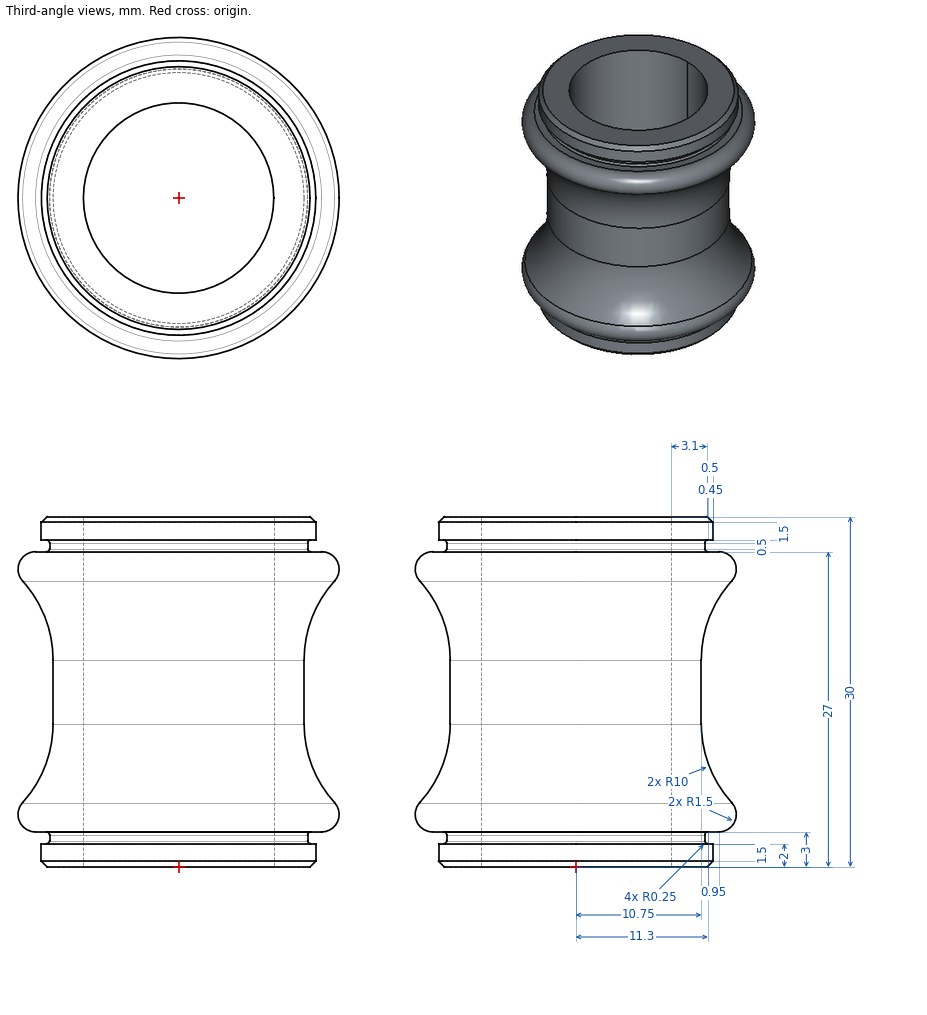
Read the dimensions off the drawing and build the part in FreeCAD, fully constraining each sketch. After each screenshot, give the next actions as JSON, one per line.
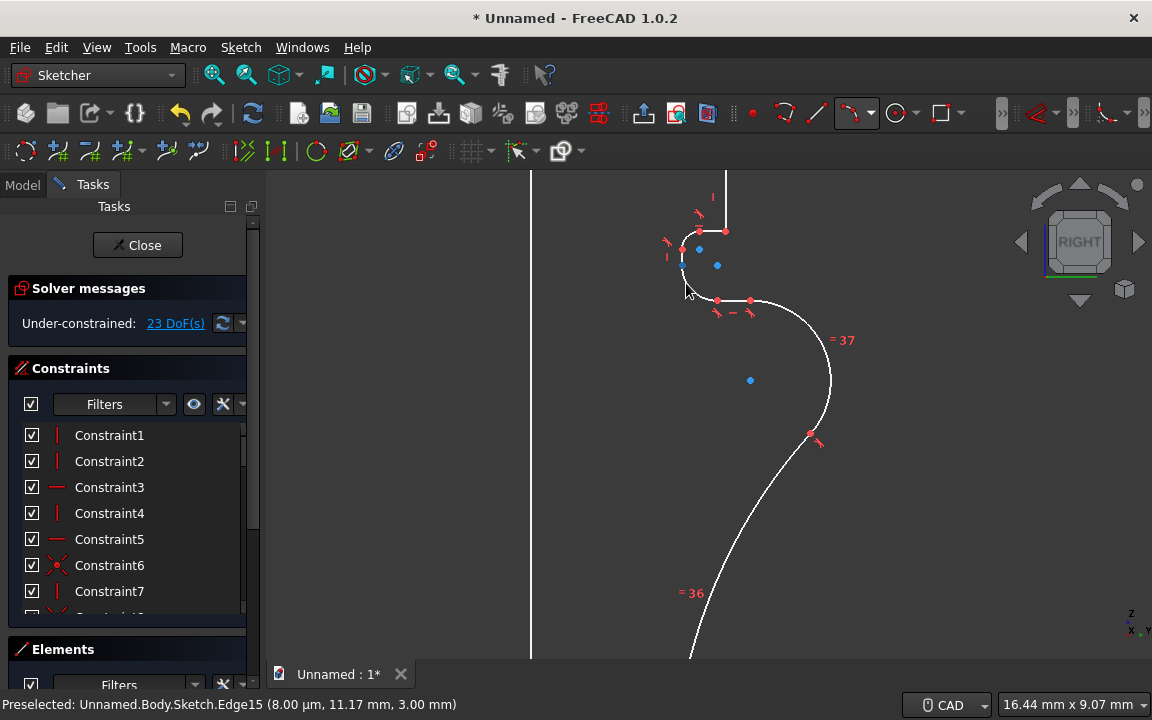
{"action": "left_click", "coordinate": [686, 282]}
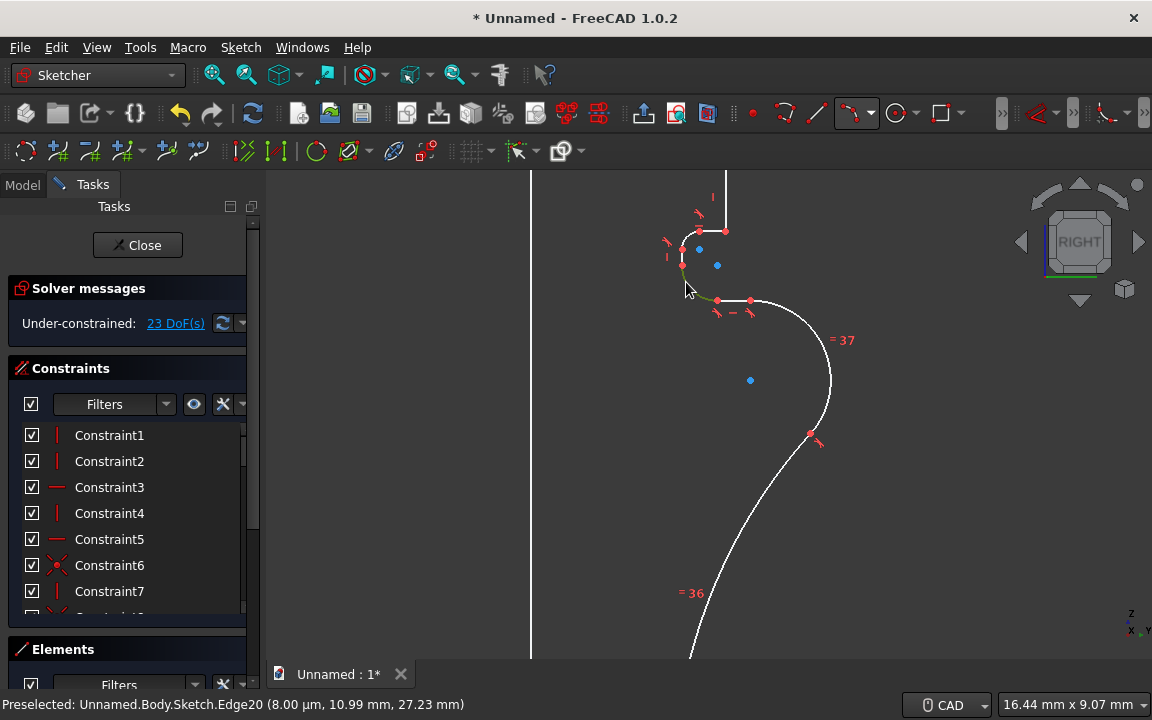
{"action": "left_click", "coordinate": [687, 237]}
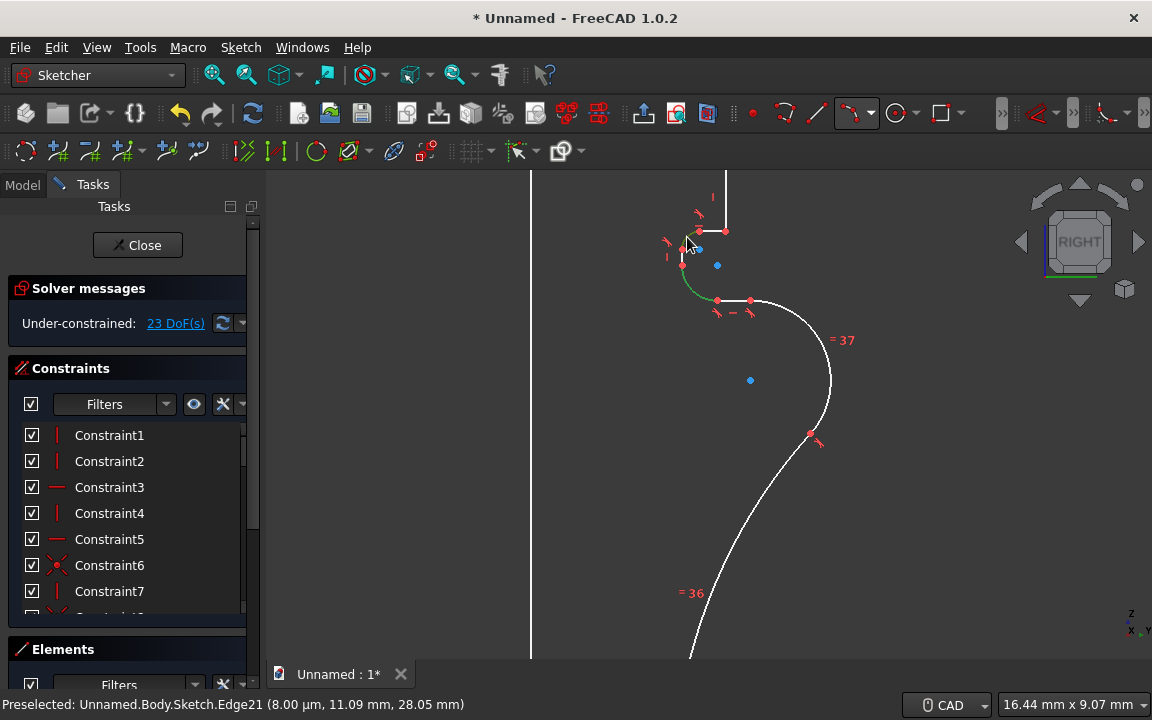
{"action": "scroll", "coordinate": [686, 282], "scroll_direction": "down", "scroll_amount": 8}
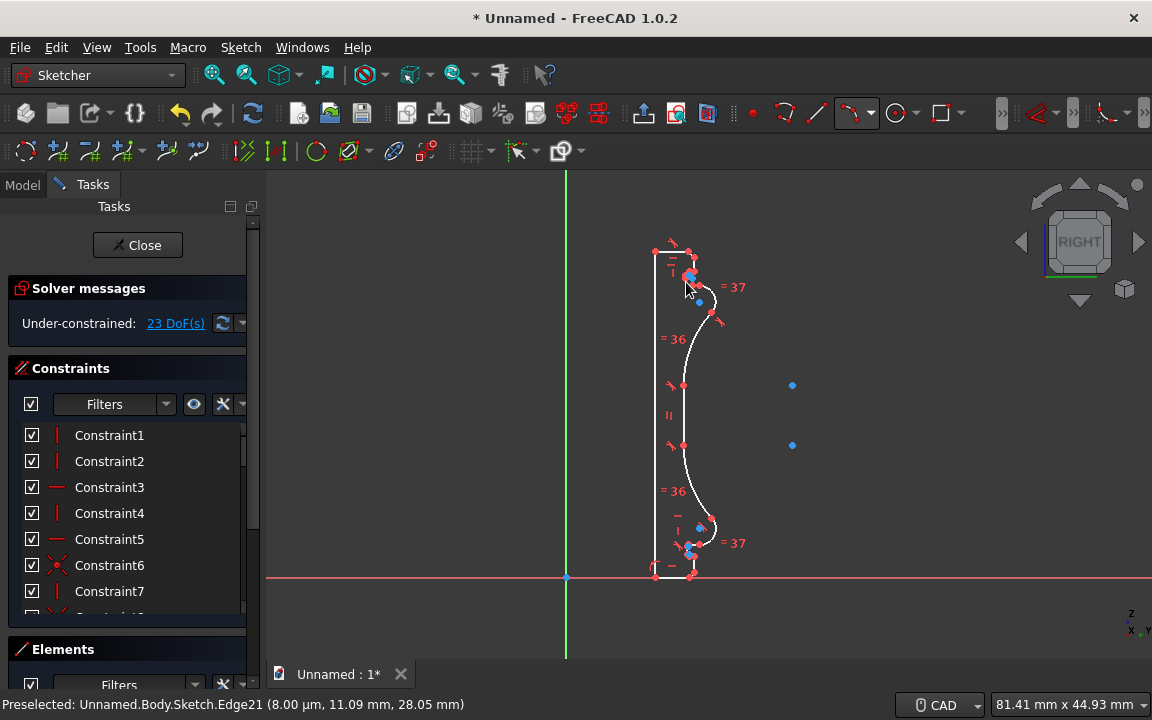
{"action": "scroll", "coordinate": [688, 556], "scroll_direction": "up", "scroll_amount": 11}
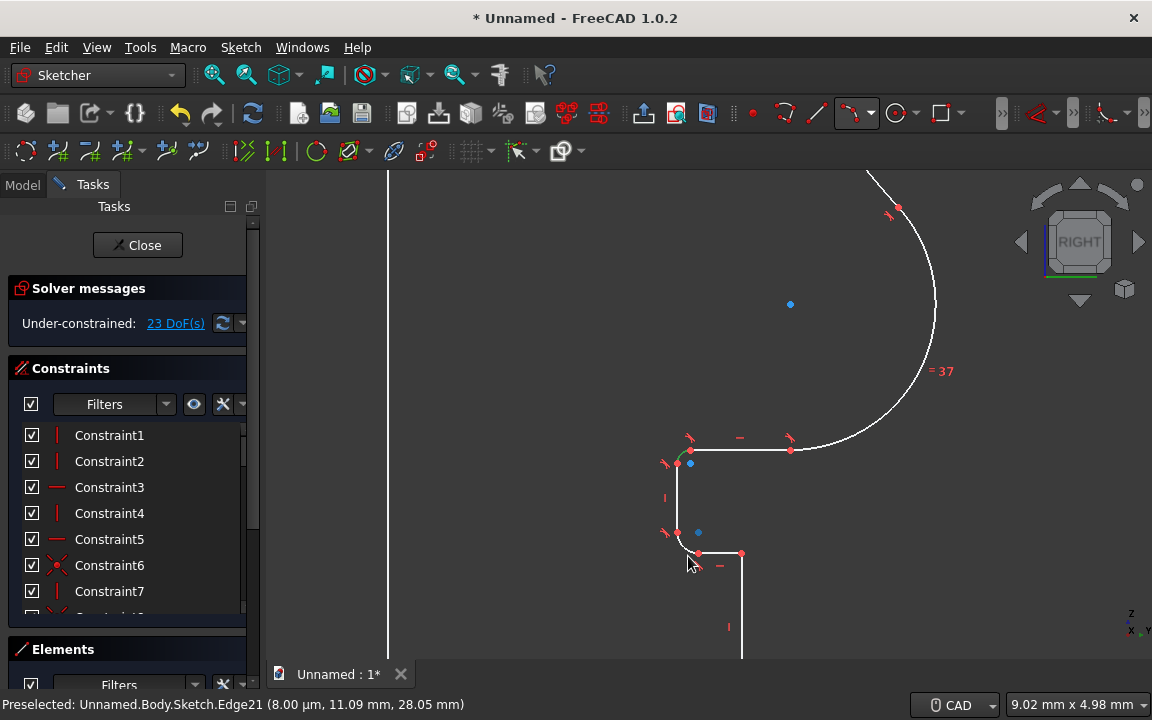
{"action": "left_click", "coordinate": [684, 547]}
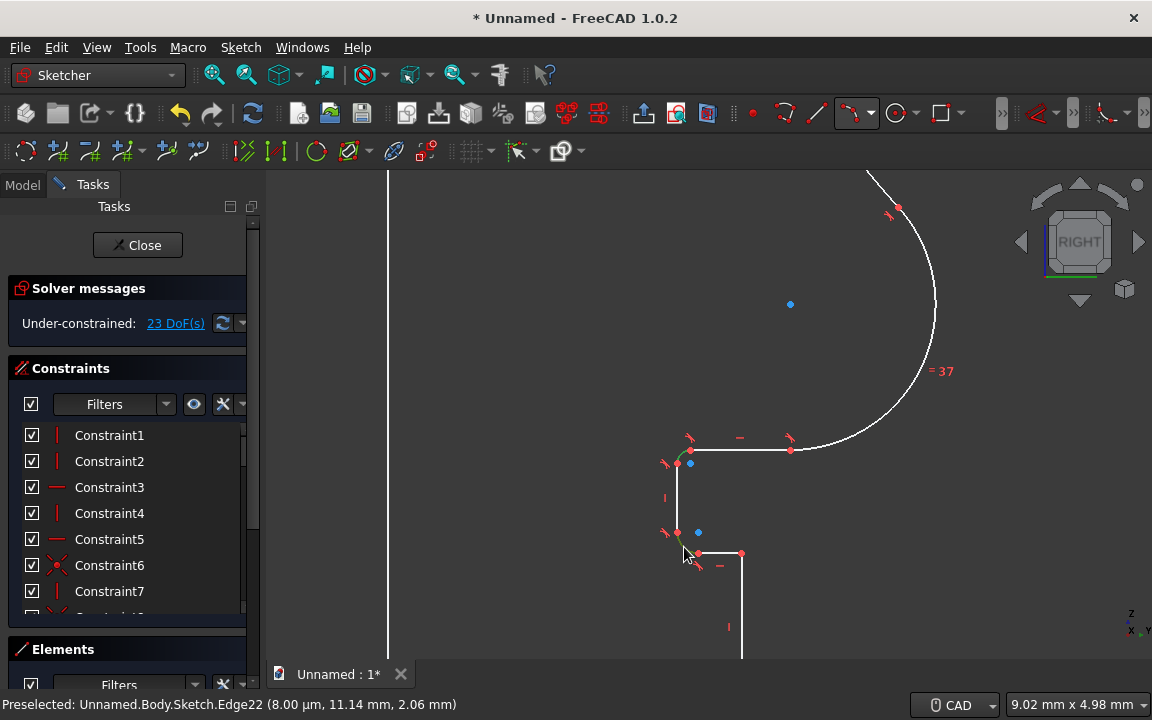
{"action": "key", "text": "e"}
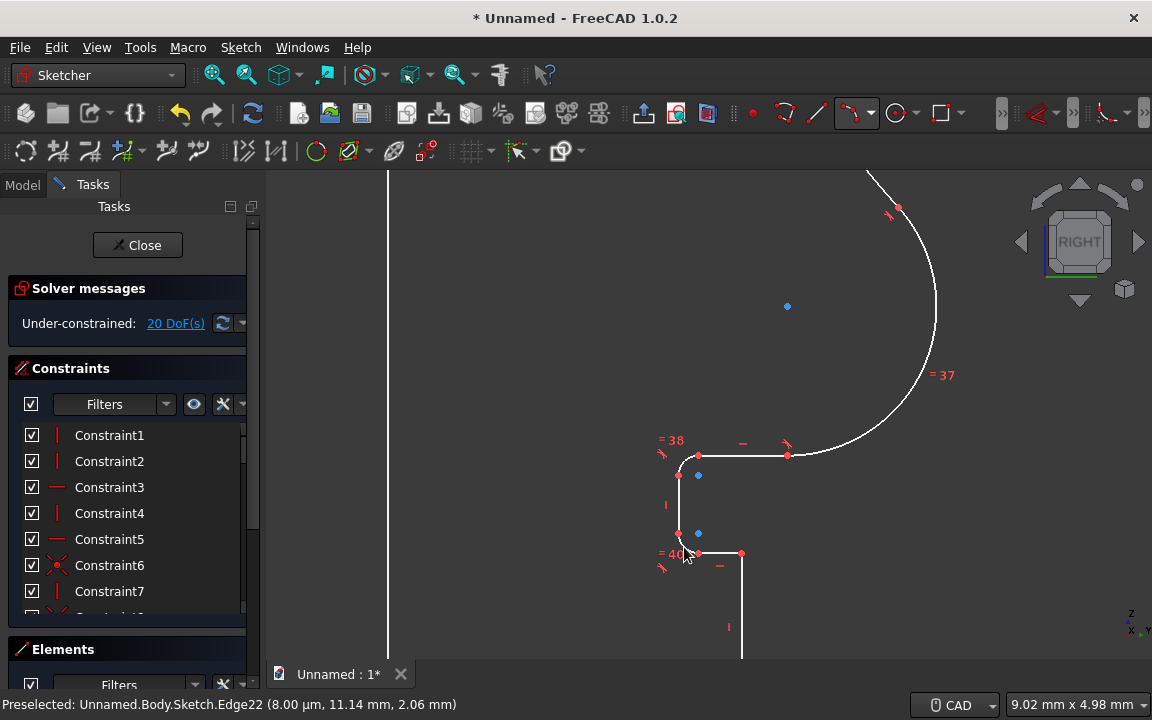
{"action": "left_click", "coordinate": [1036, 114]}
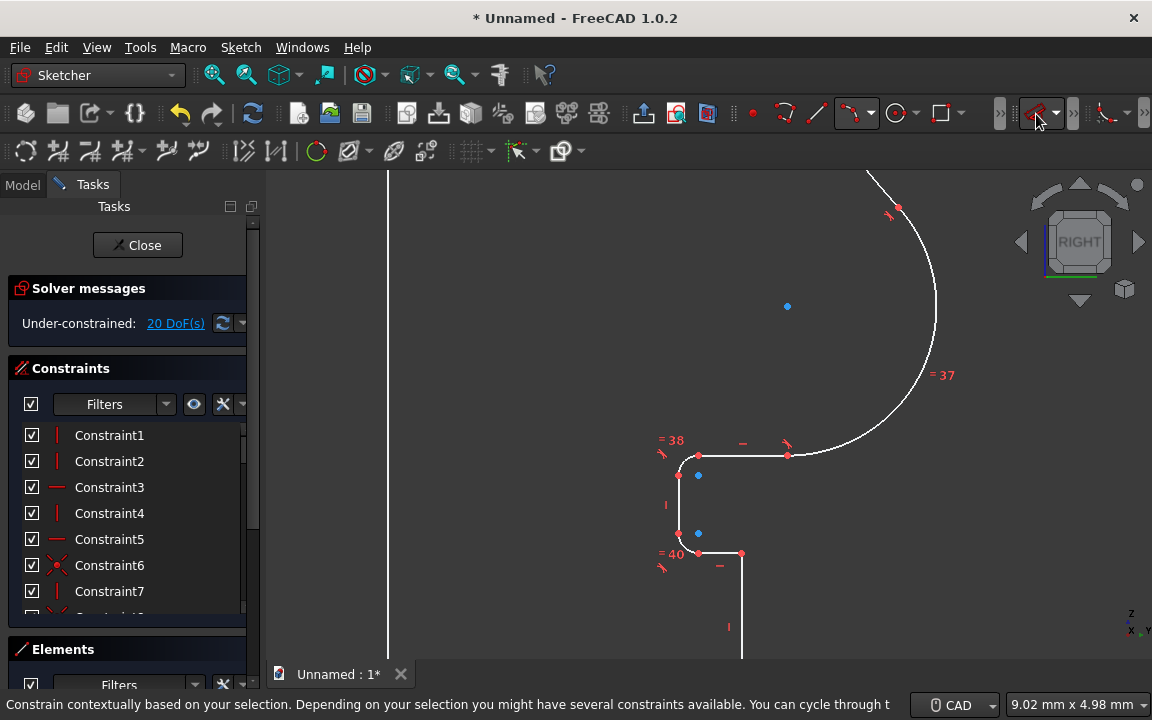
{"action": "scroll", "coordinate": [689, 458], "scroll_direction": "up", "scroll_amount": 3}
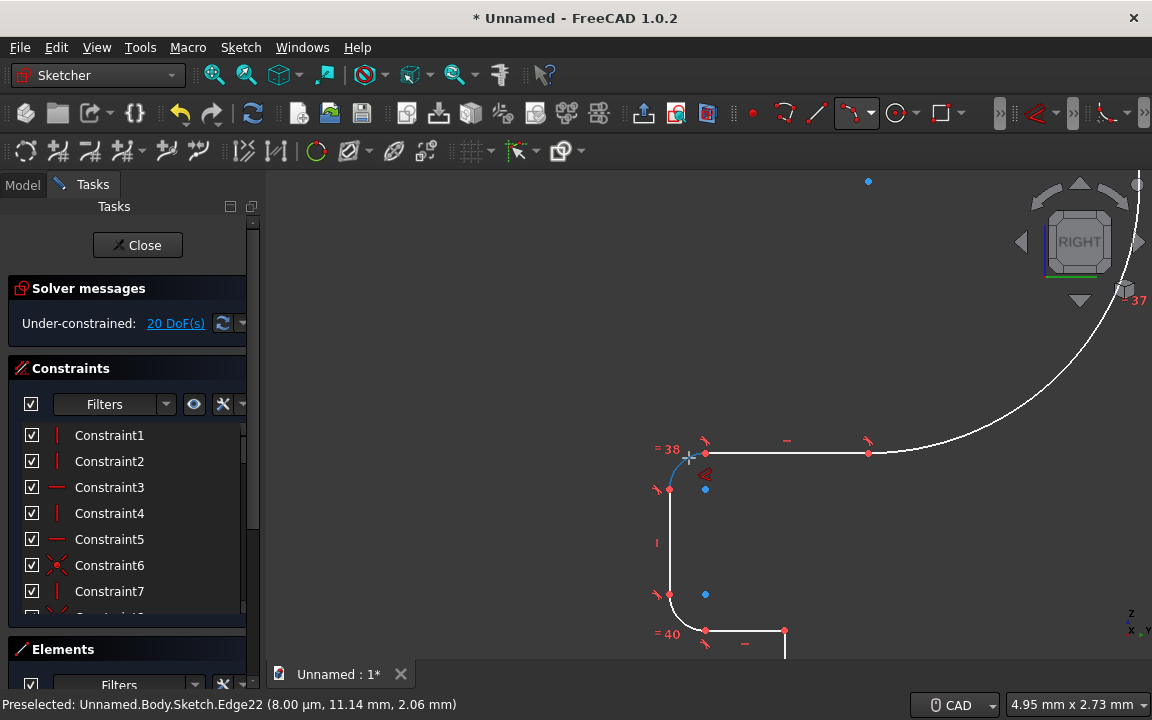
{"action": "left_click", "coordinate": [689, 457]}
{"action": "left_click", "coordinate": [674, 429]}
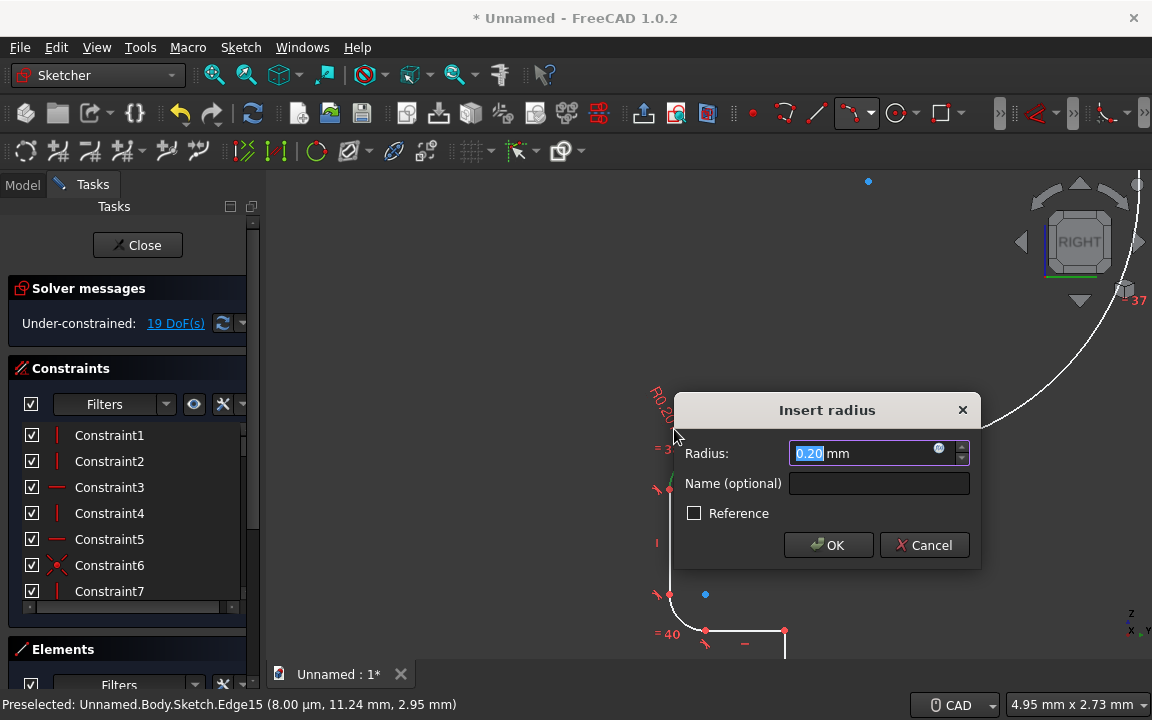
{"action": "type", "text": "0.25"}
{"action": "key", "text": "Return"}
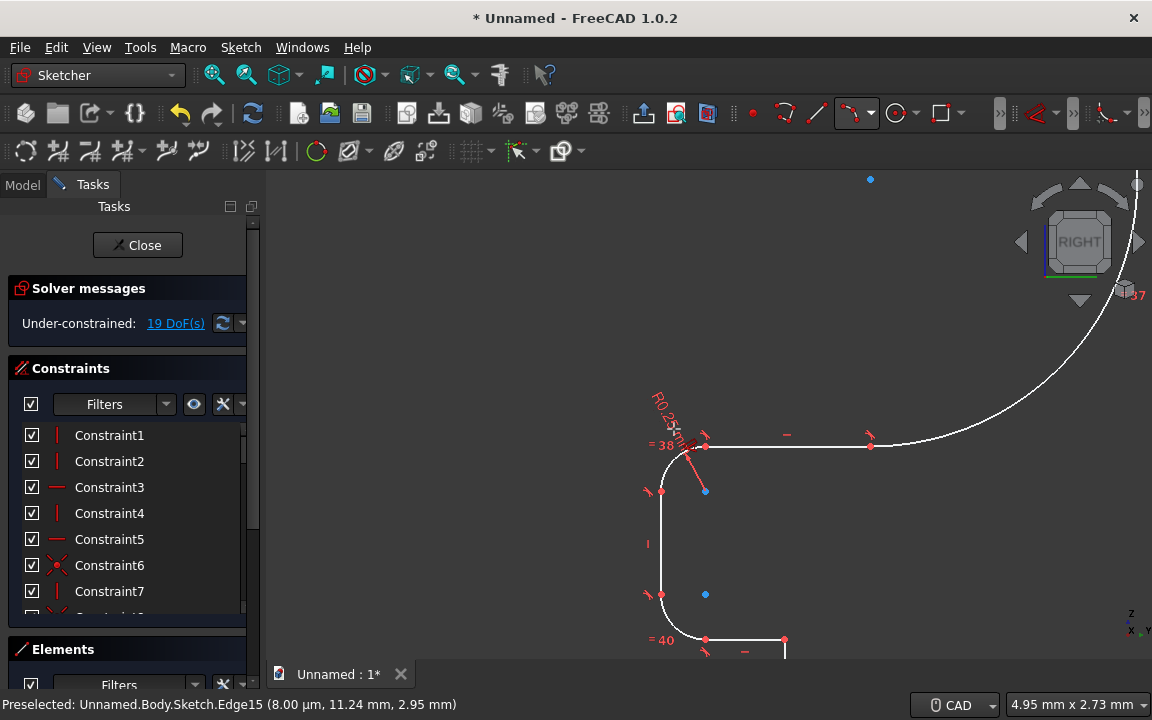
{"action": "scroll", "coordinate": [688, 551], "scroll_direction": "down", "scroll_amount": 14}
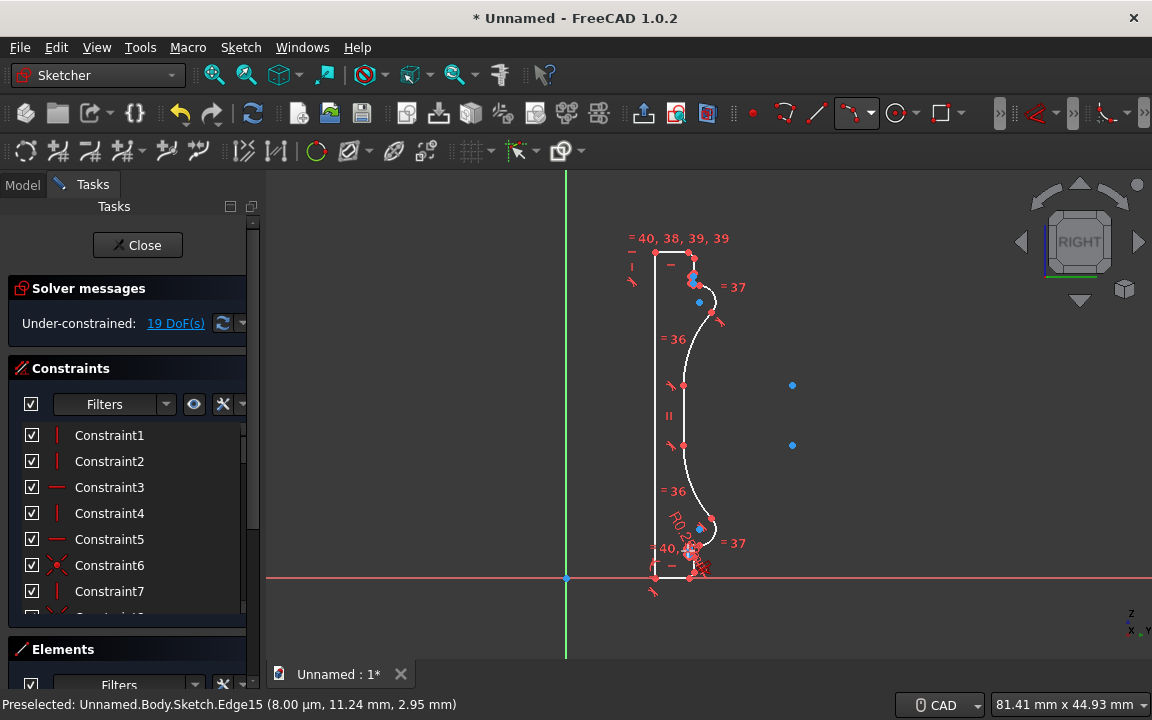
{"action": "scroll", "coordinate": [710, 542], "scroll_direction": "up", "scroll_amount": 5}